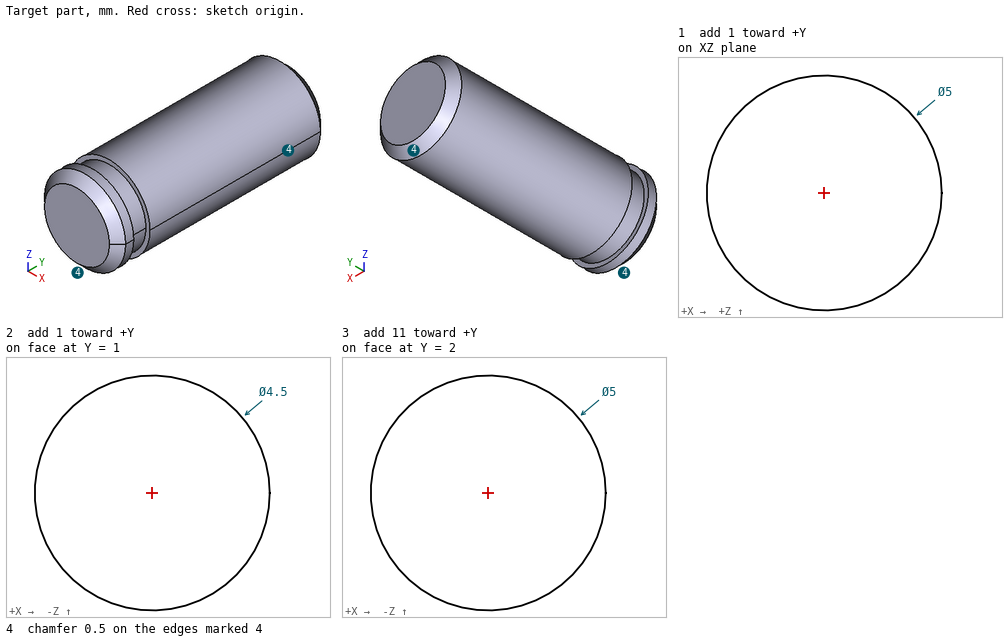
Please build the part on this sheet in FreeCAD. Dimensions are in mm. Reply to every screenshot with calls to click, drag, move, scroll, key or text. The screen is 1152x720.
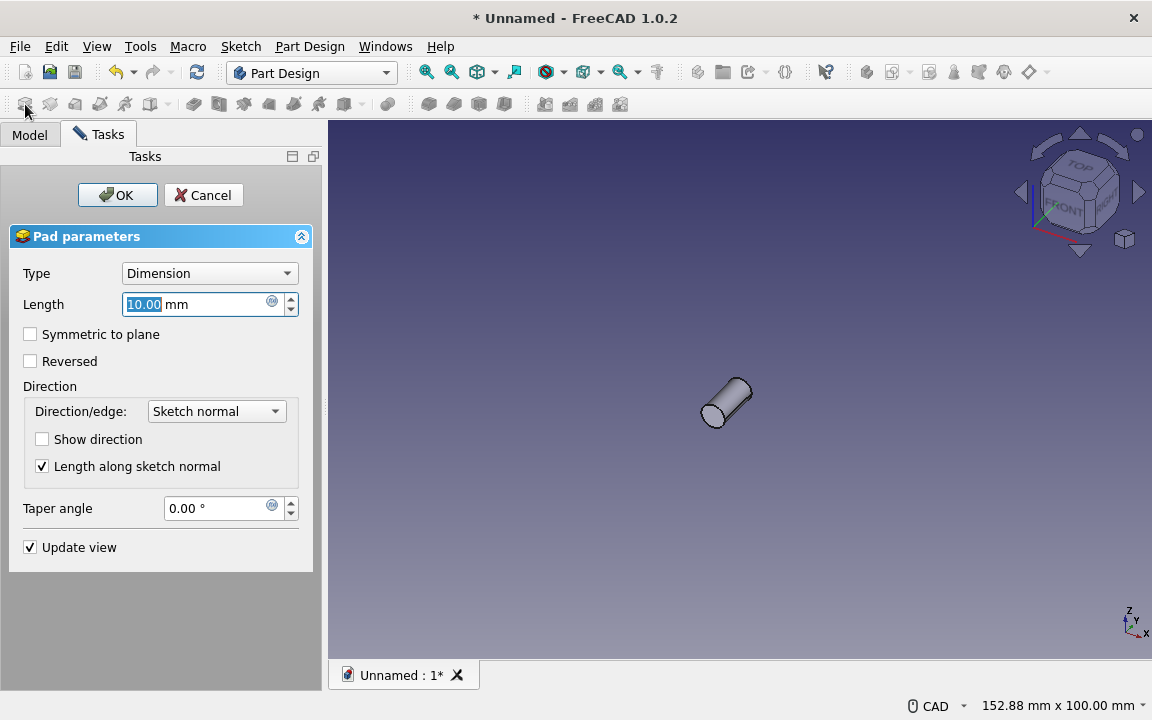
text(1)
key(Tab)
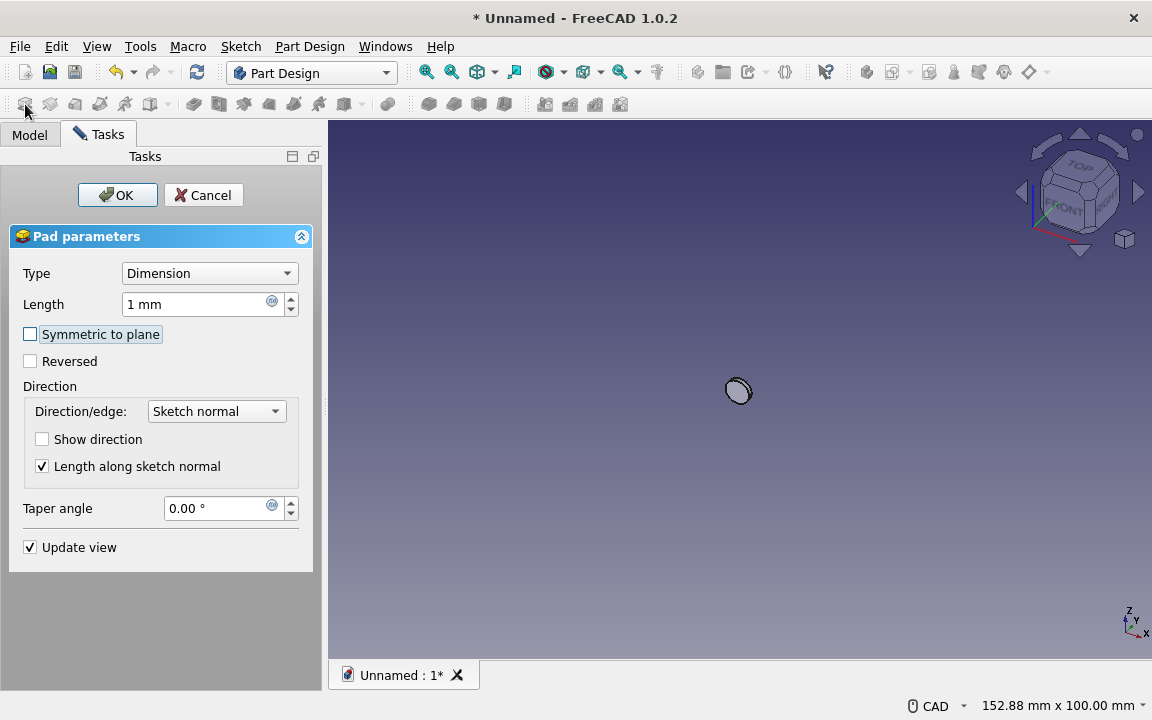
click(31, 361)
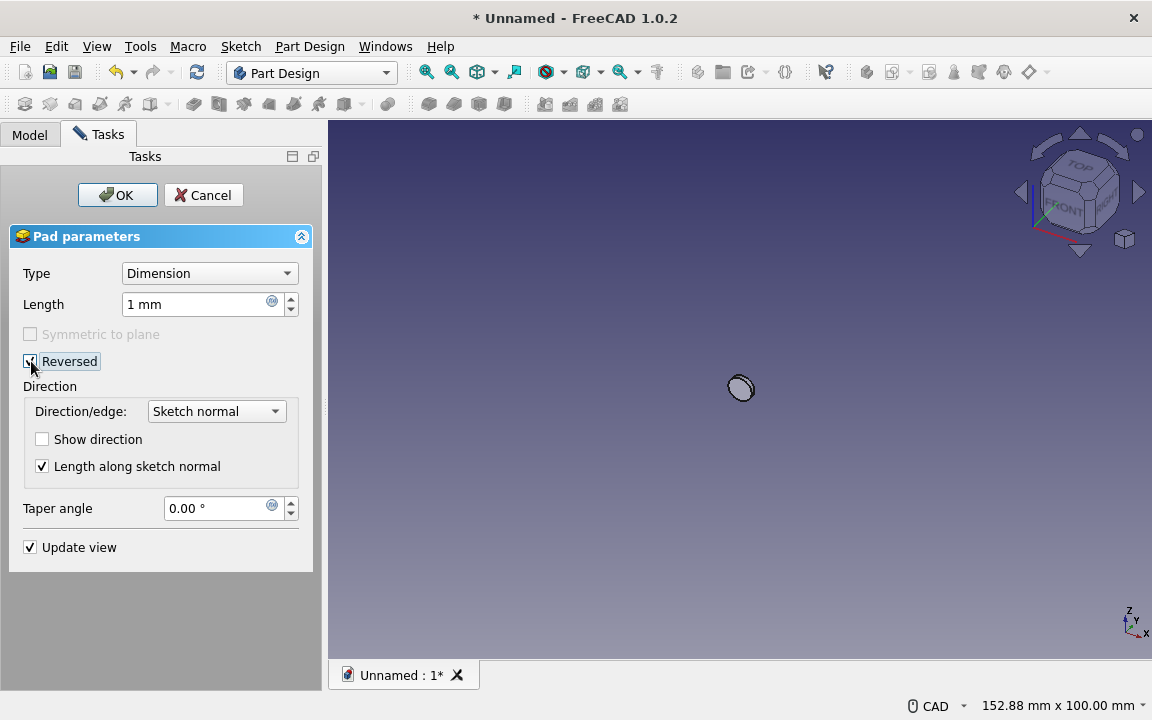
click(118, 195)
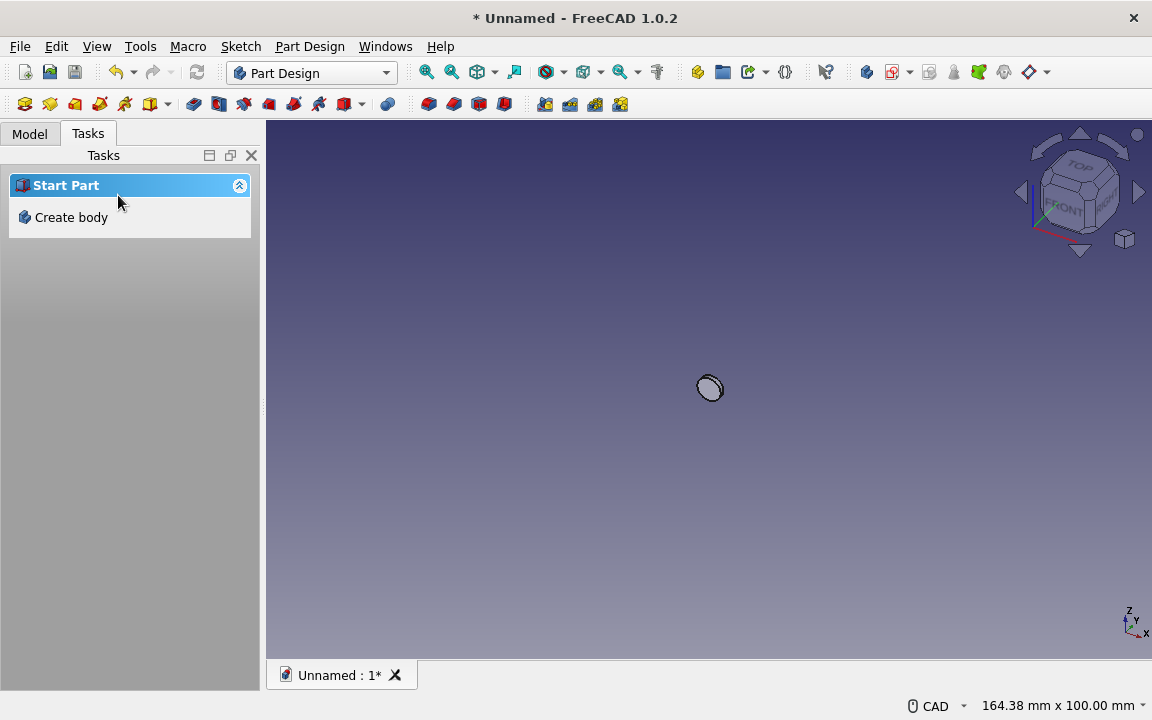
key(v)
key(f)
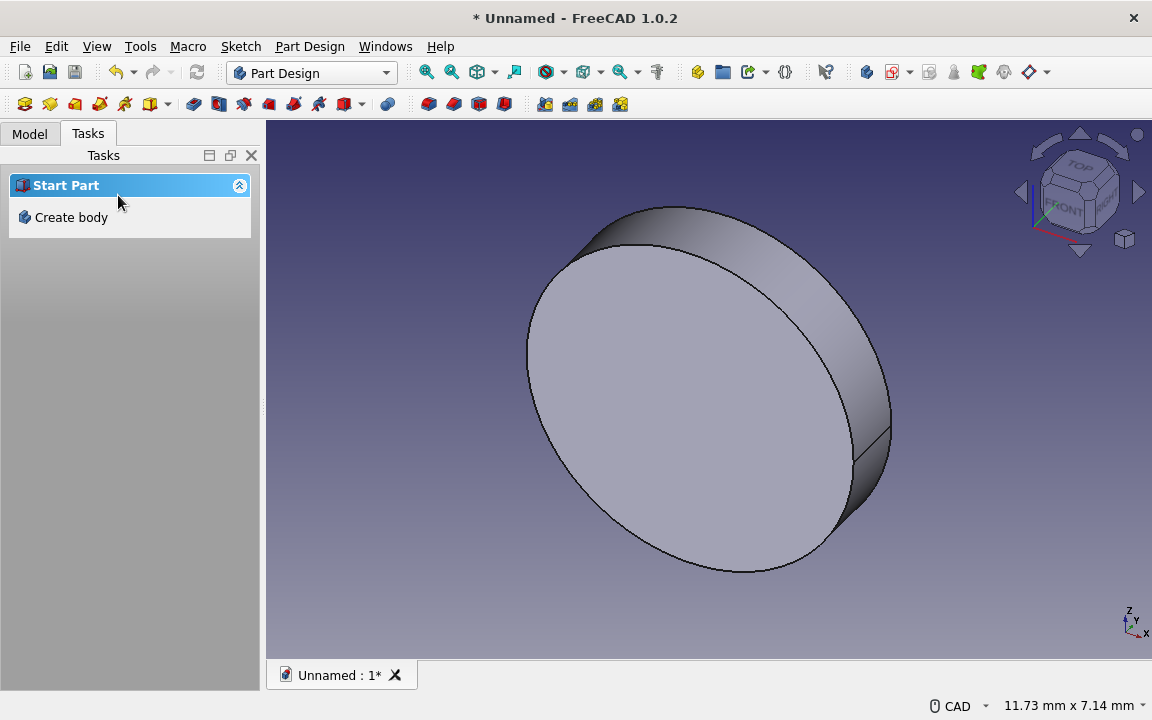
key(4)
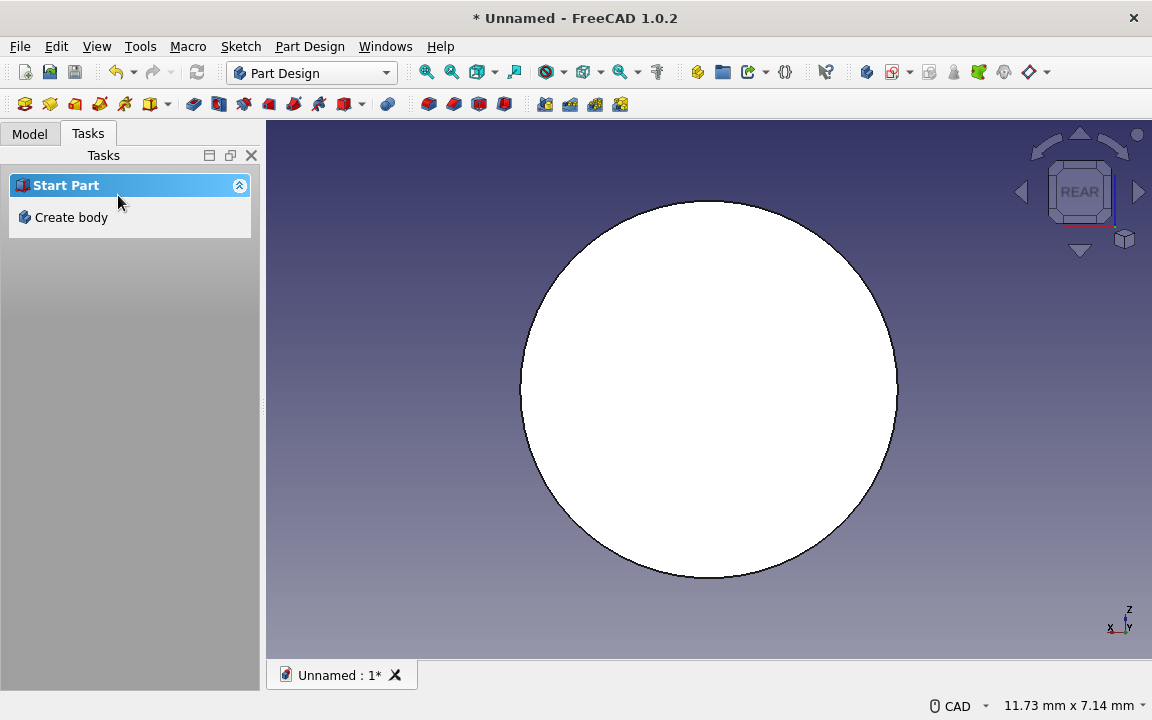
click(709, 389)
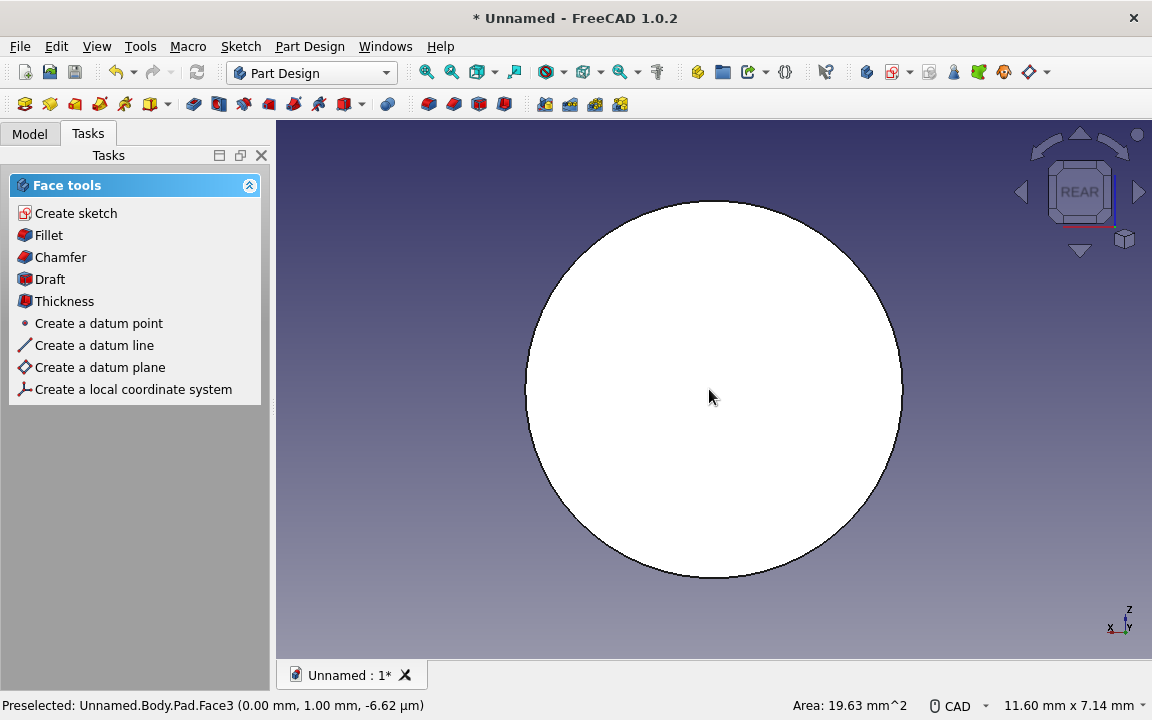
click(892, 72)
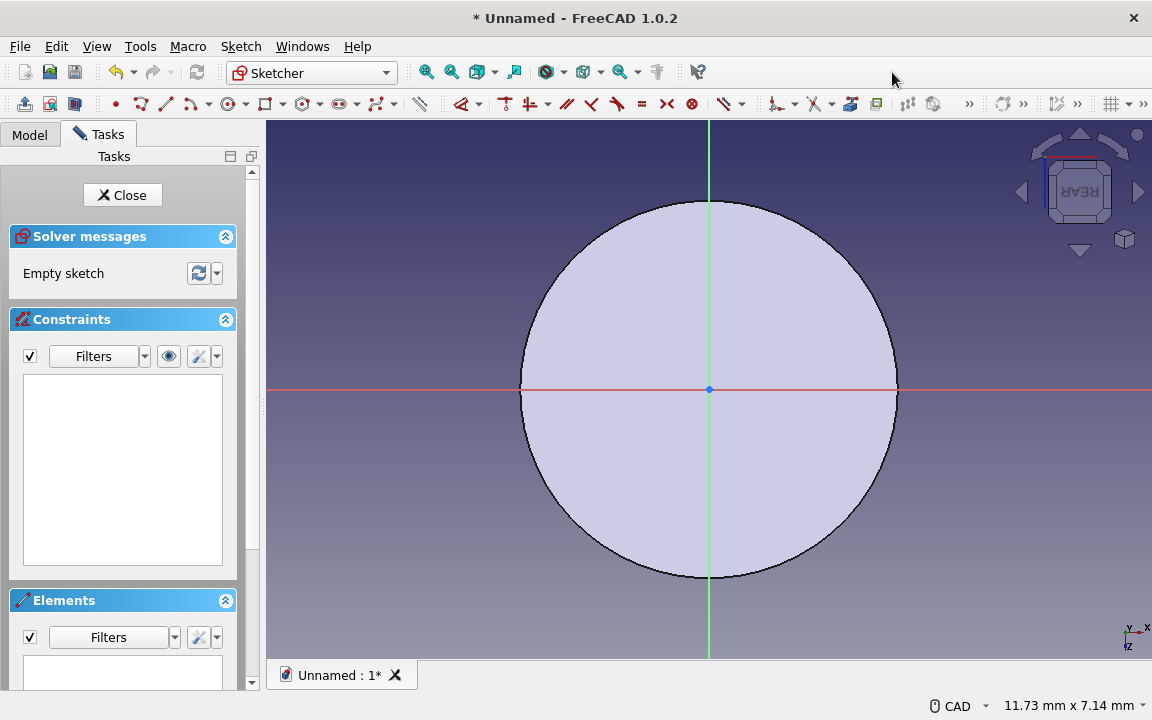
key(g)
key(c)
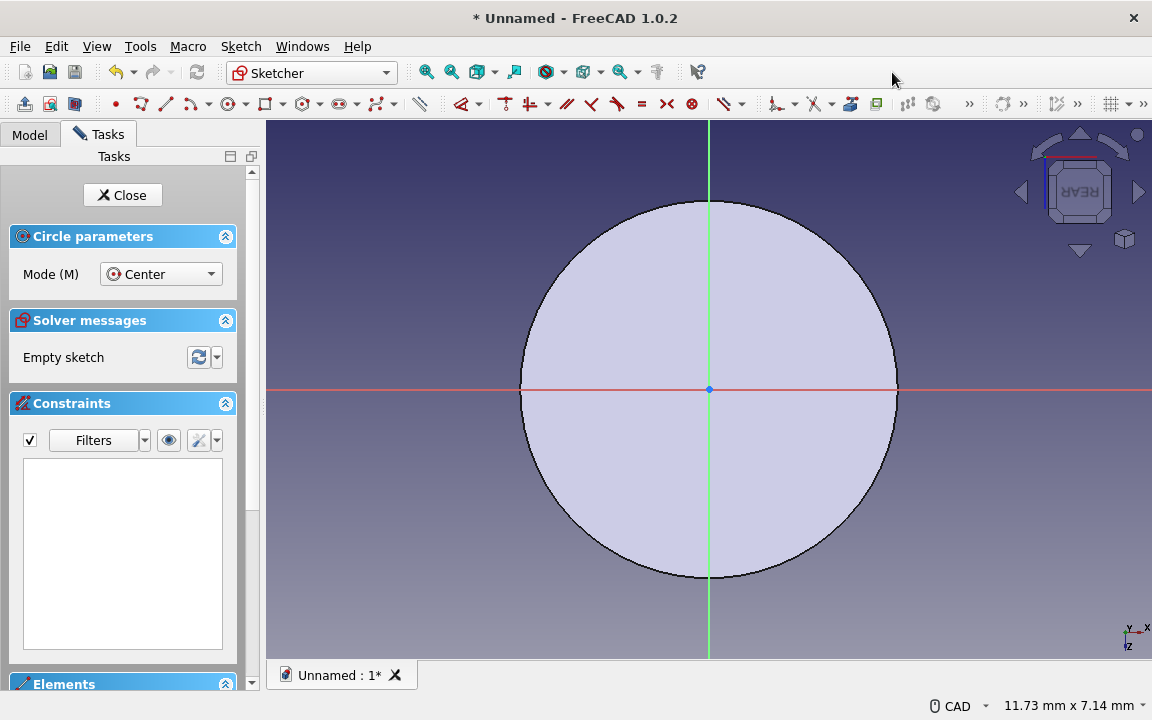
click(709, 389)
click(829, 269)
key(Escape)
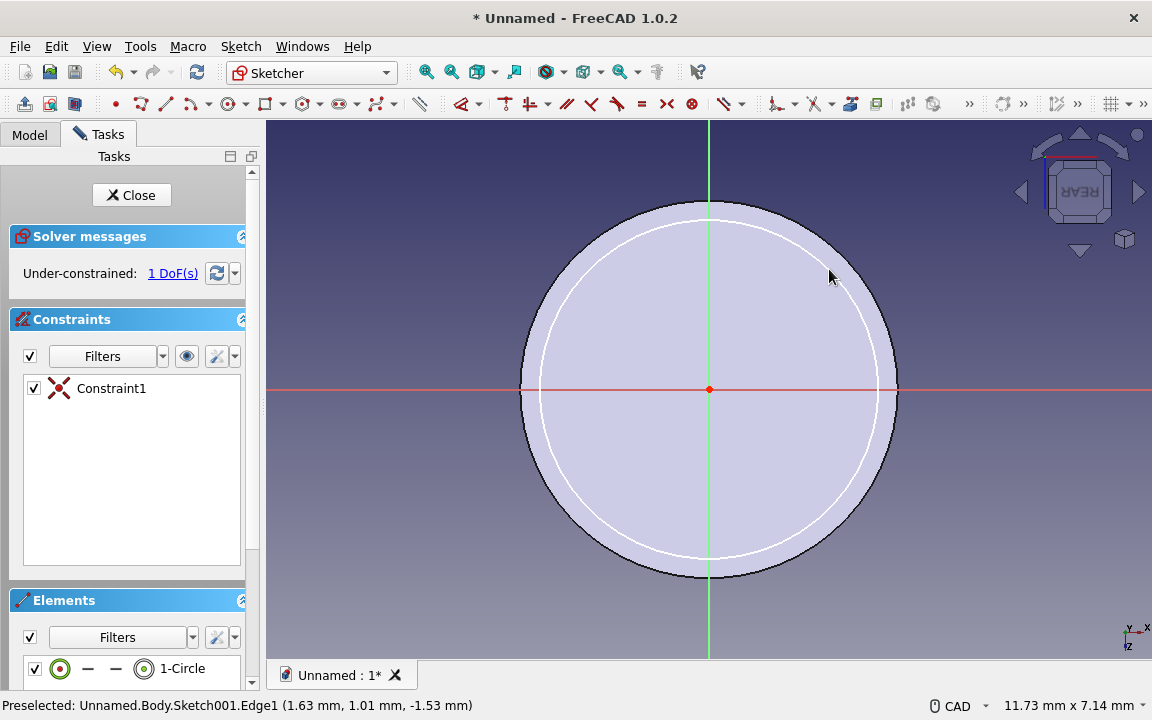
key(d)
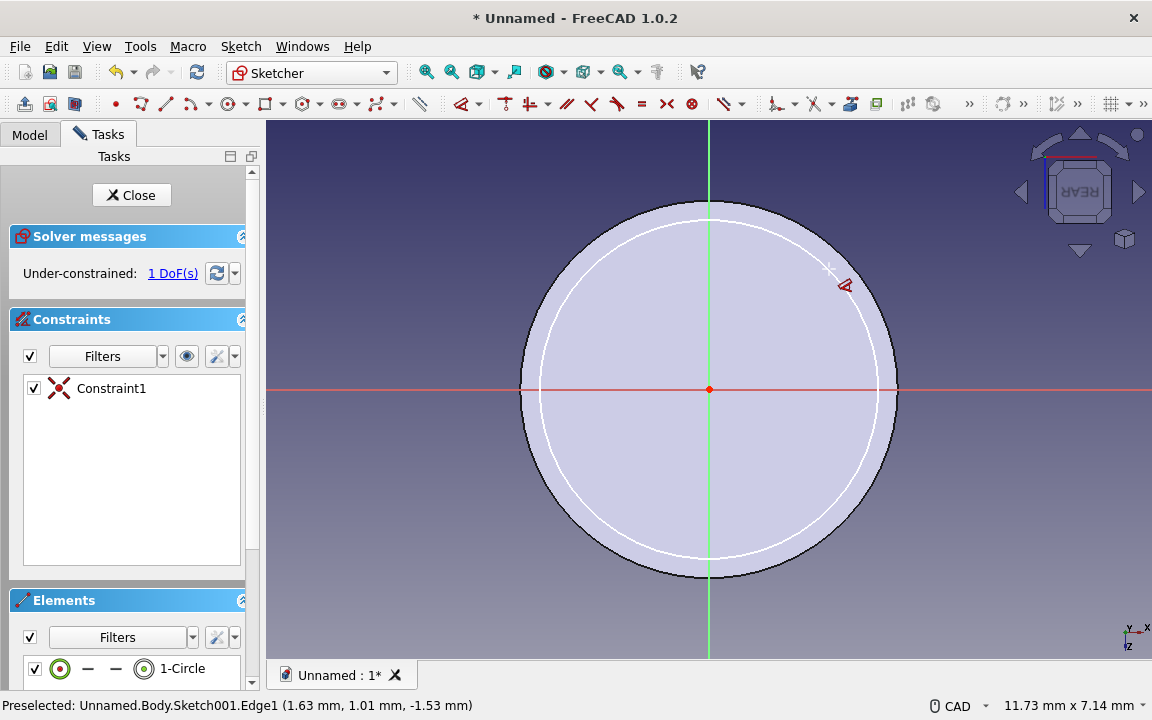
click(828, 269)
click(850, 246)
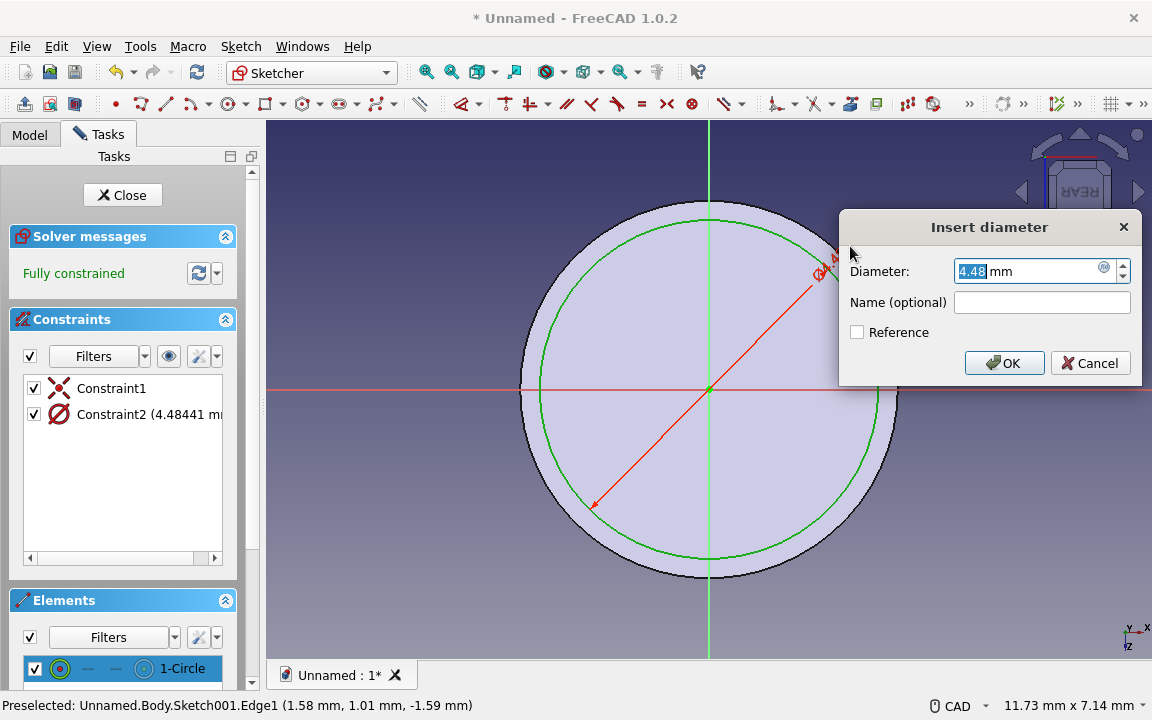
text(4.5)
key(Return)
key(Escape)